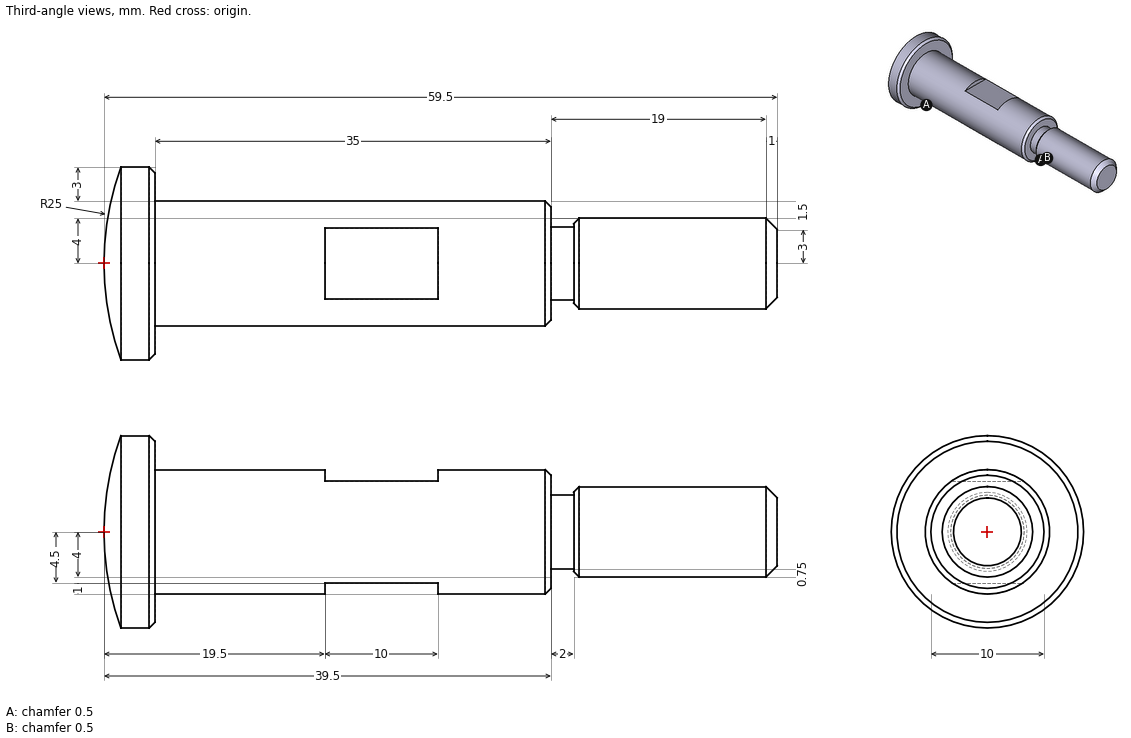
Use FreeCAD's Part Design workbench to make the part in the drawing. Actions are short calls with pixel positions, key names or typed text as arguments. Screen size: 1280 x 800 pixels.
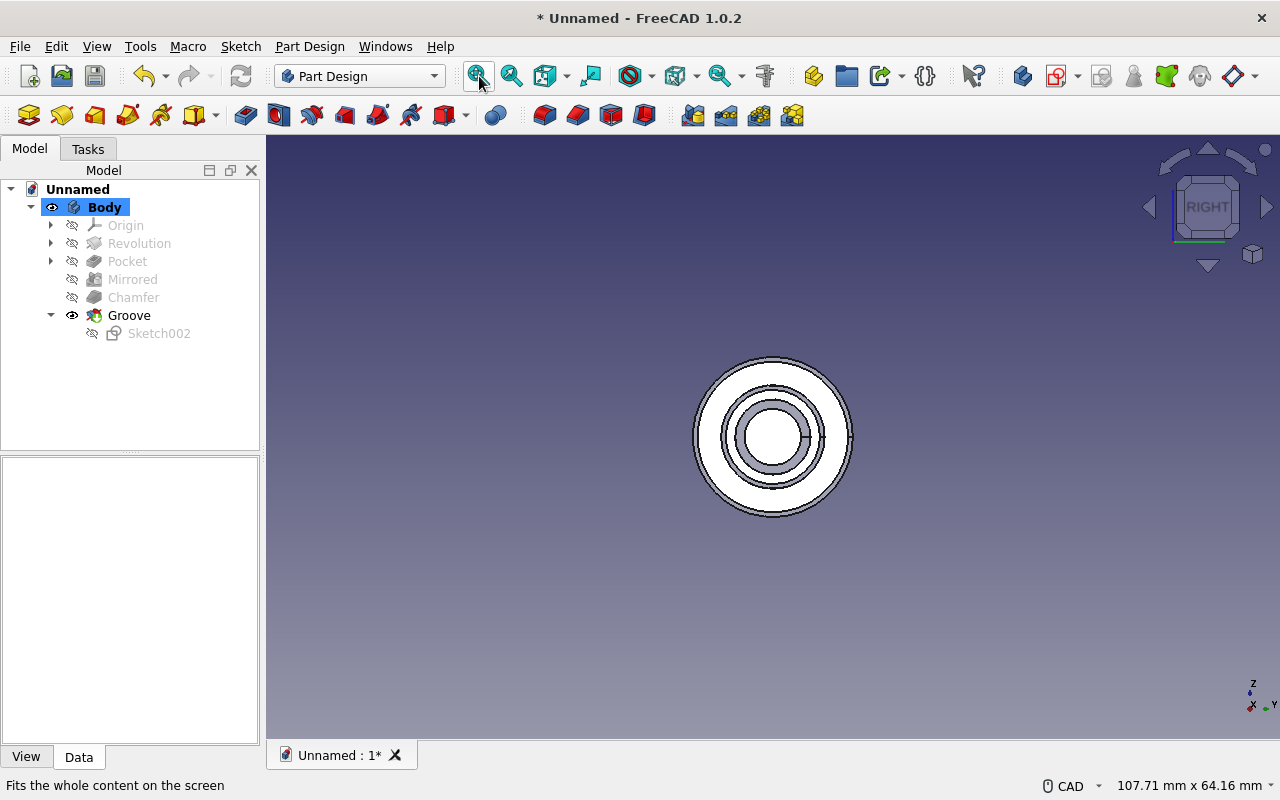
key(v)
key(f)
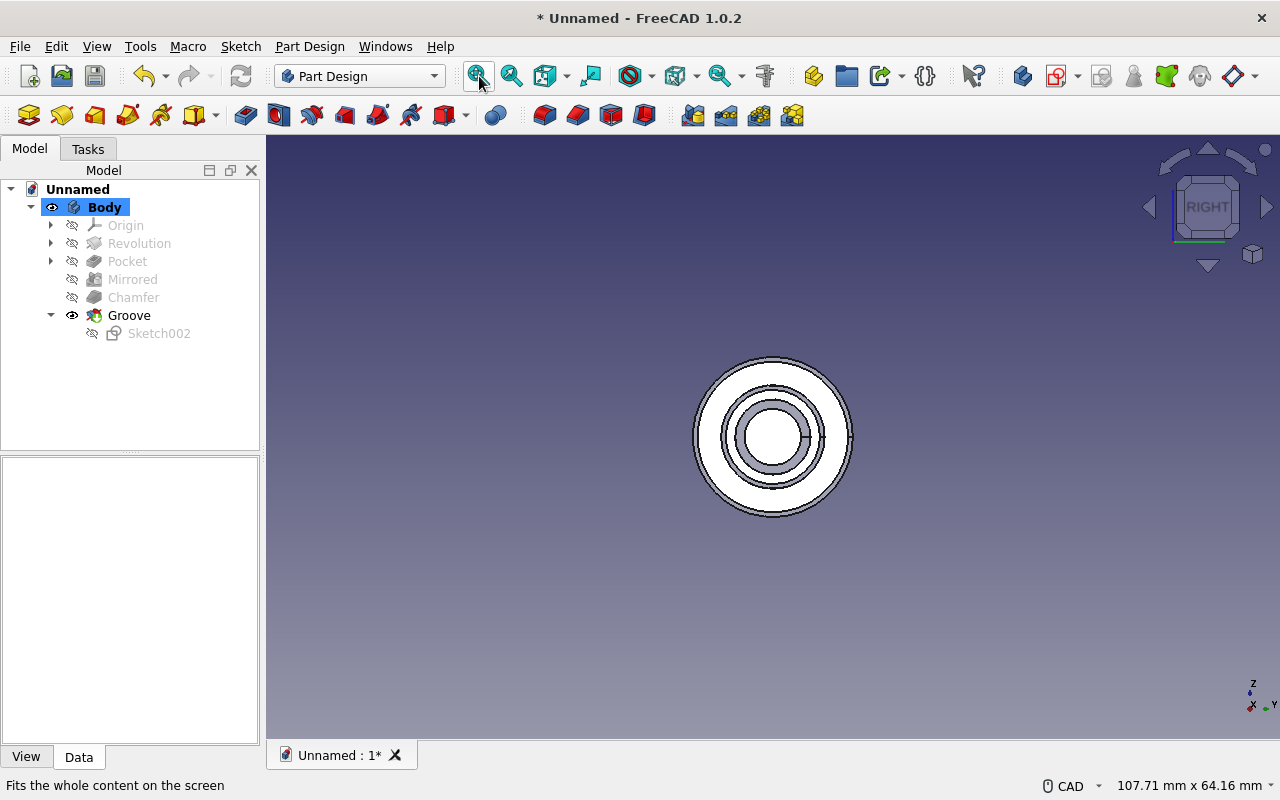
key(5)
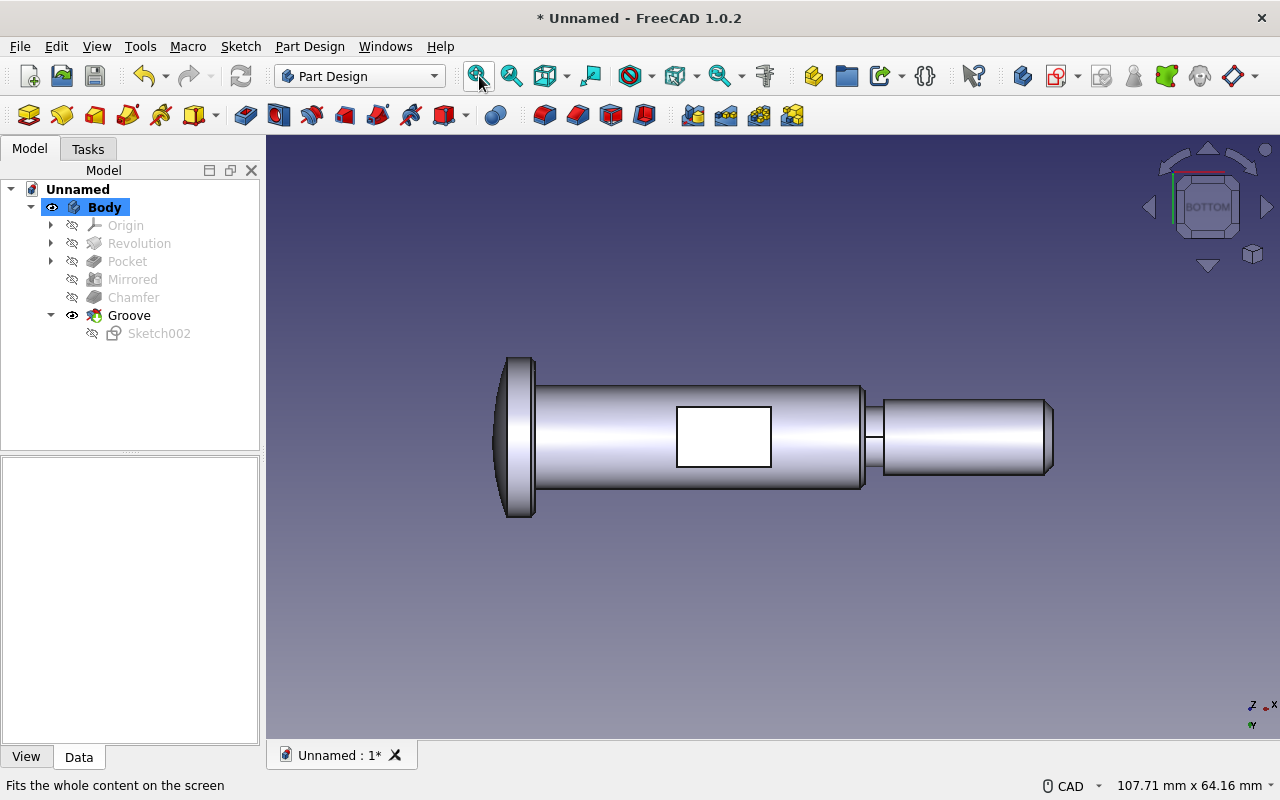
click(884, 462)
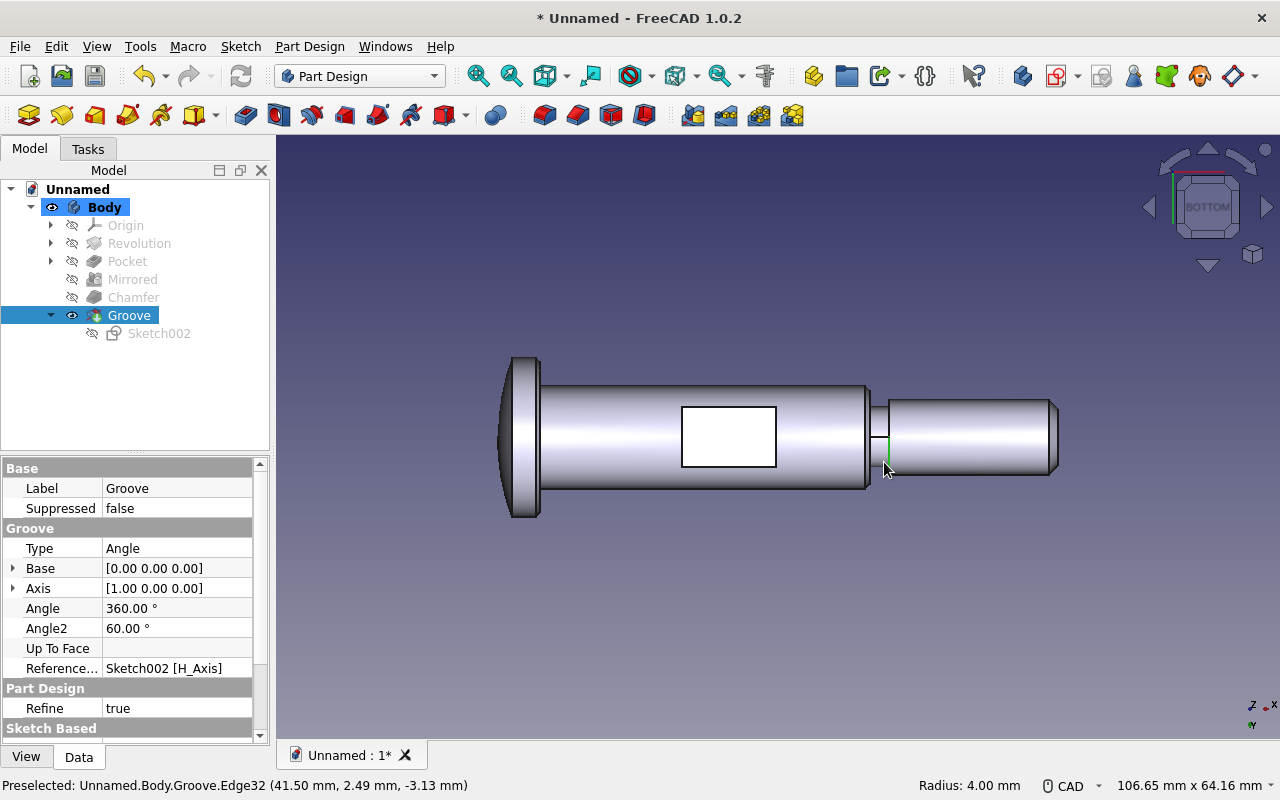
click(578, 116)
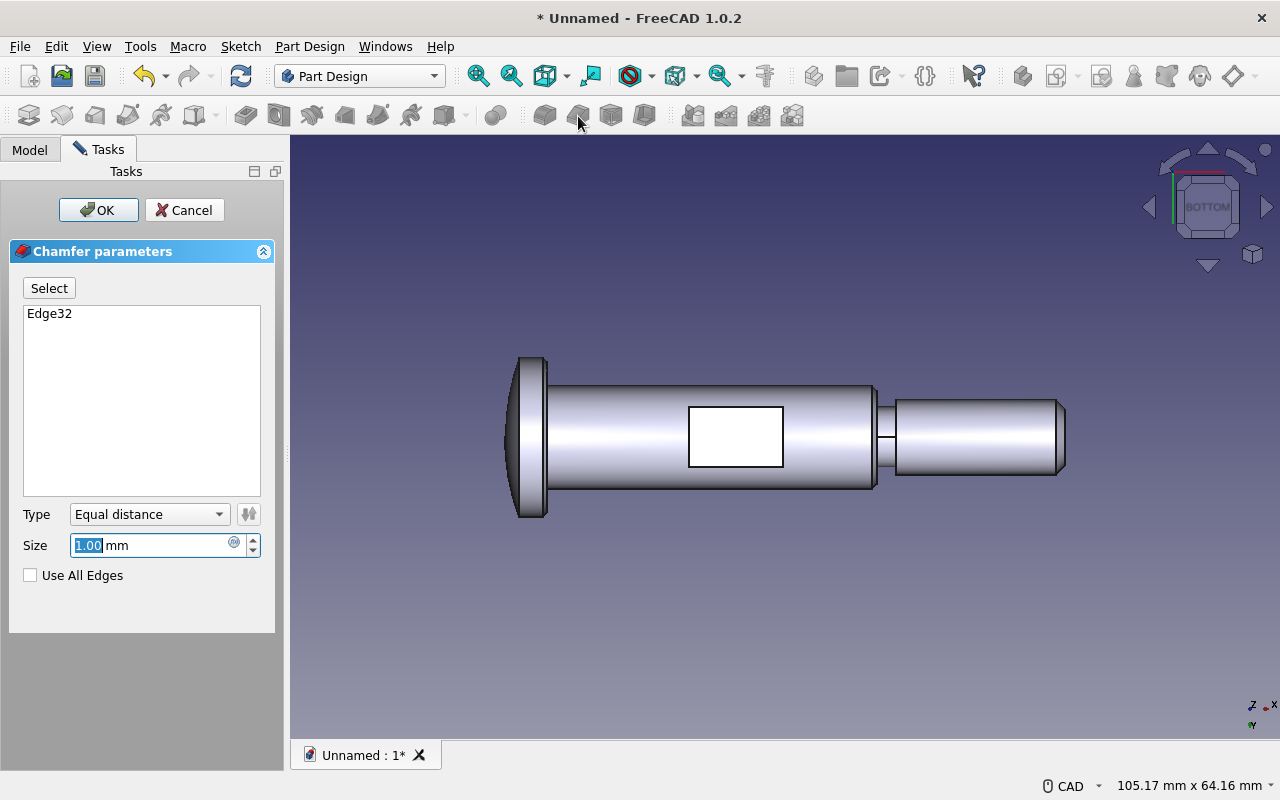
text(0.5)
key(Tab)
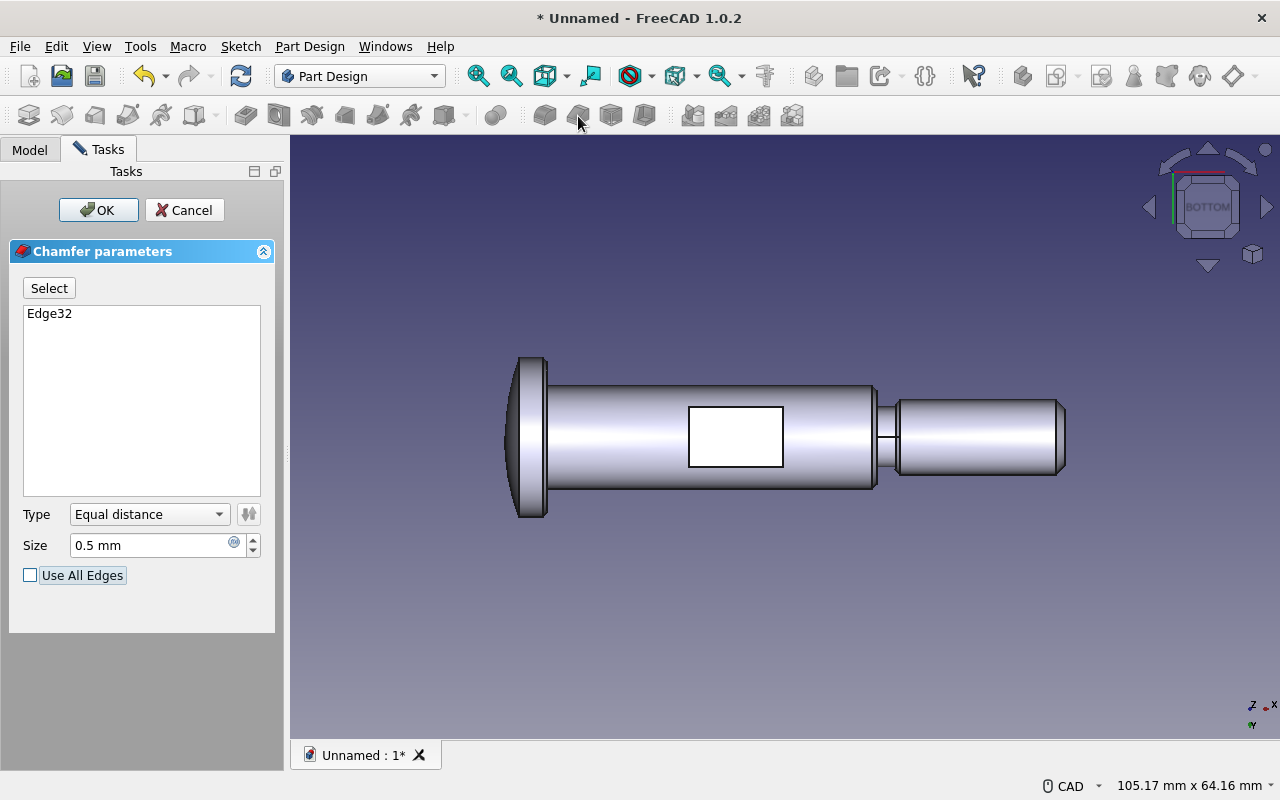
click(99, 210)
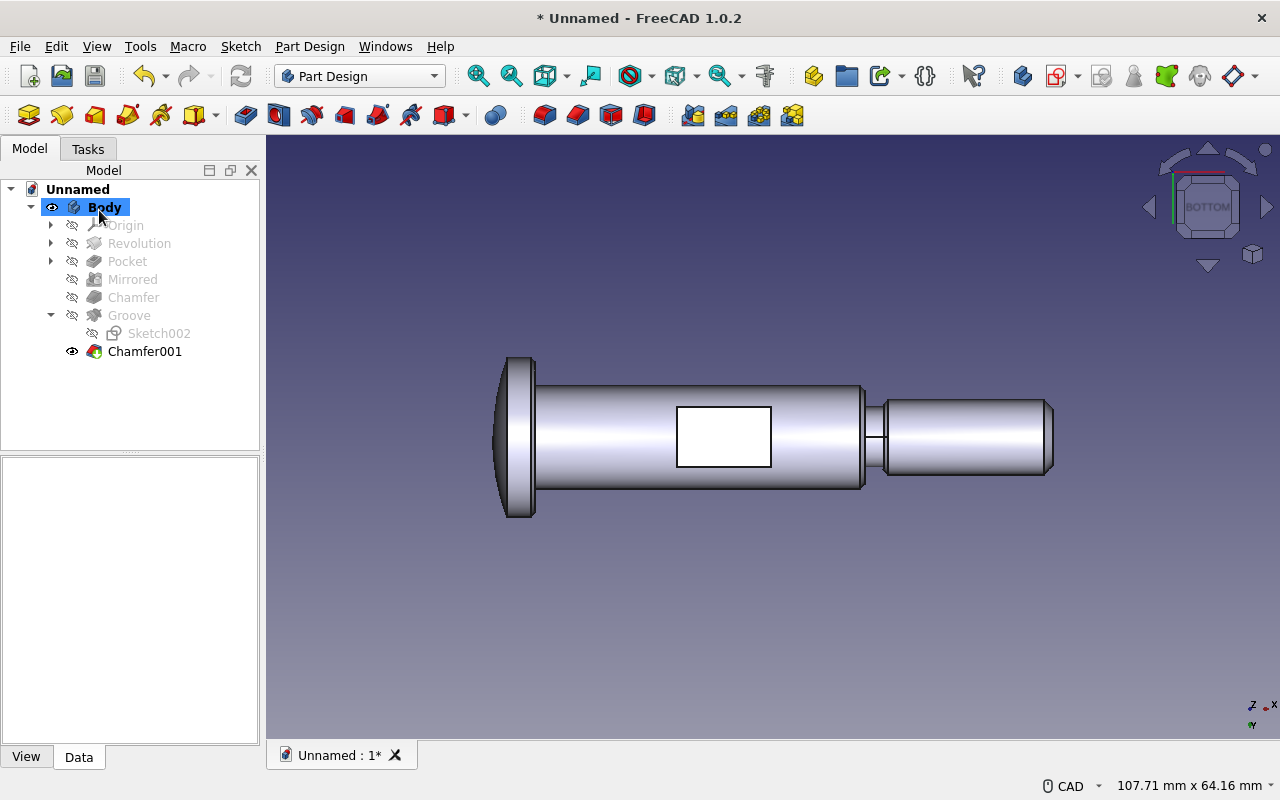
key(0)